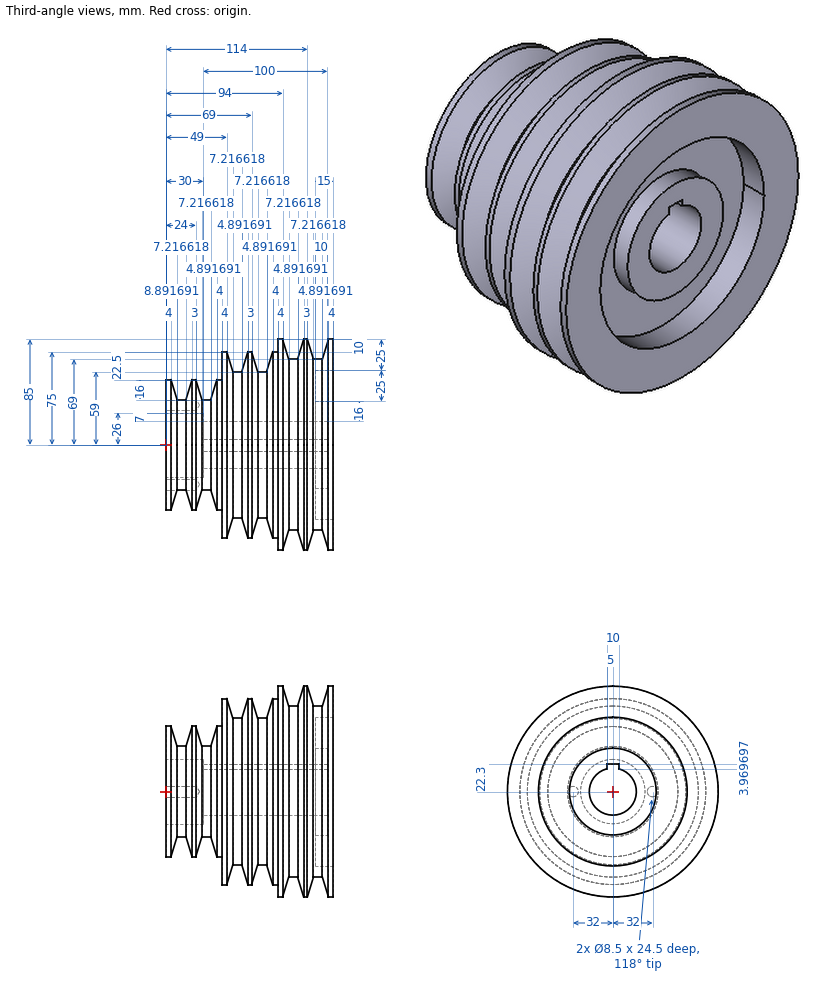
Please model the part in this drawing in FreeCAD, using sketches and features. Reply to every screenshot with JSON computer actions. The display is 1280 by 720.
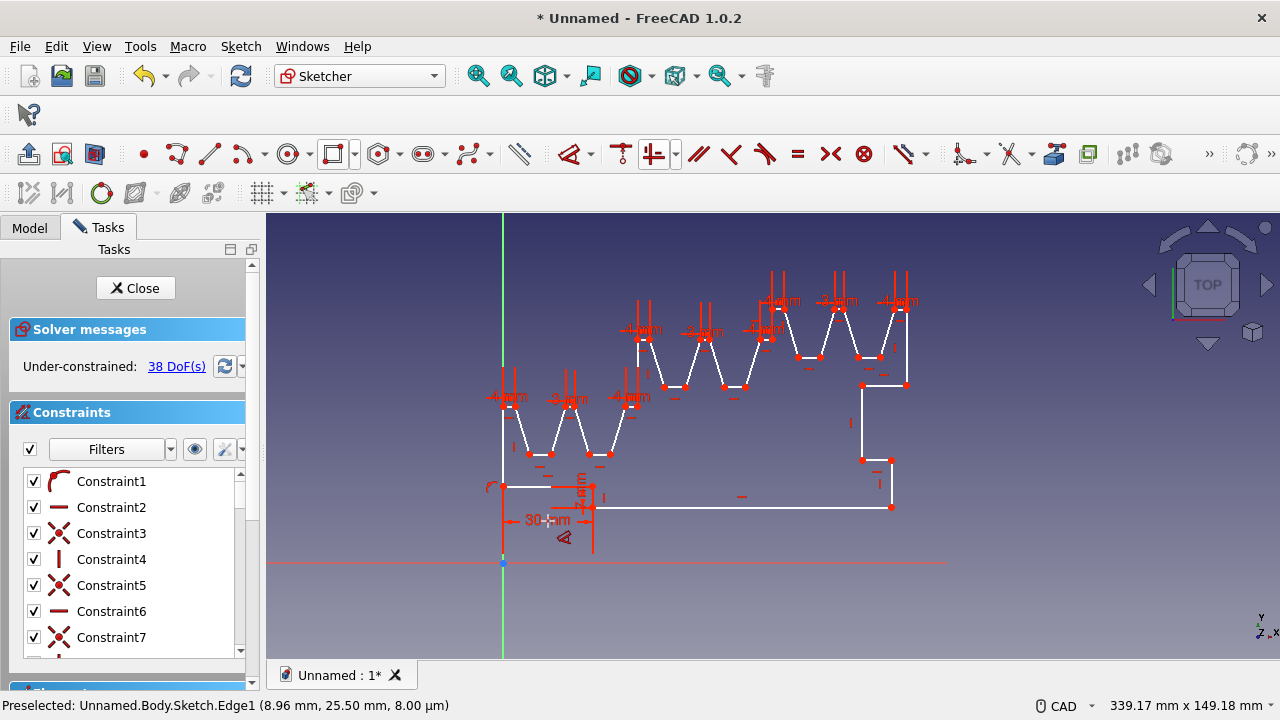
{"action": "left_click", "coordinate": [892, 494]}
{"action": "left_click", "coordinate": [926, 484]}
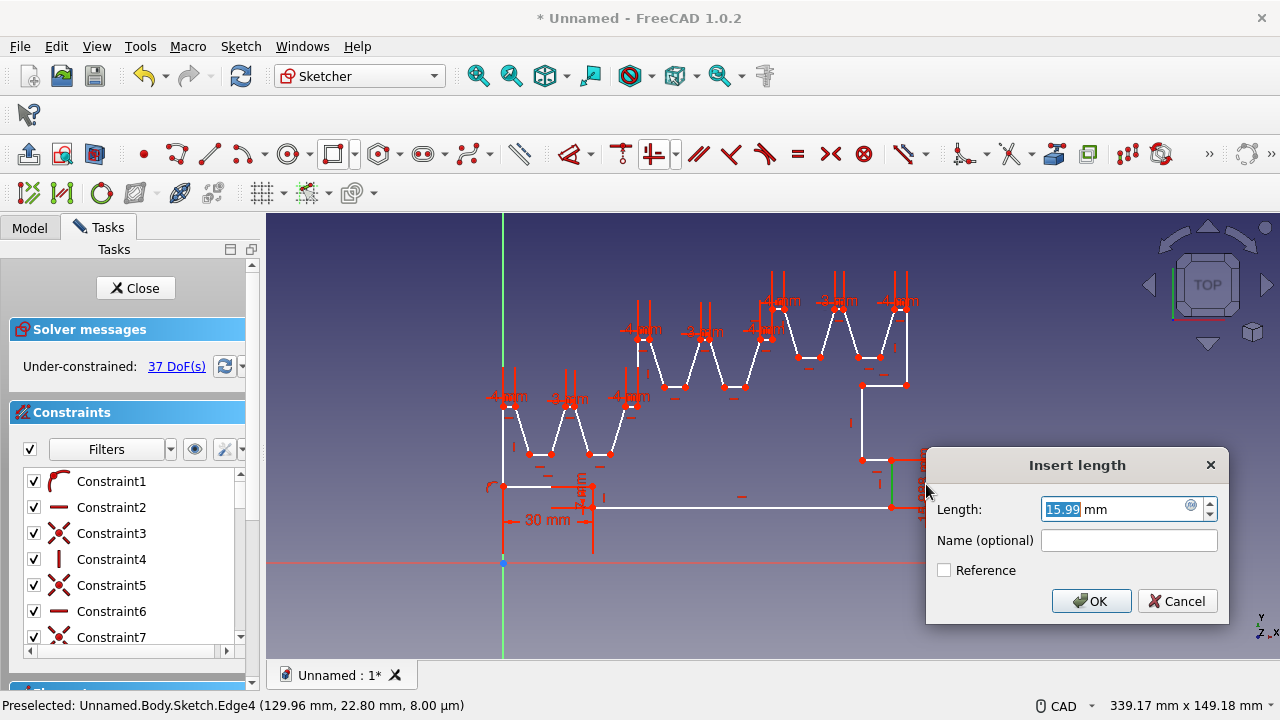
{"action": "type", "text": "16"}
{"action": "key", "text": "Return"}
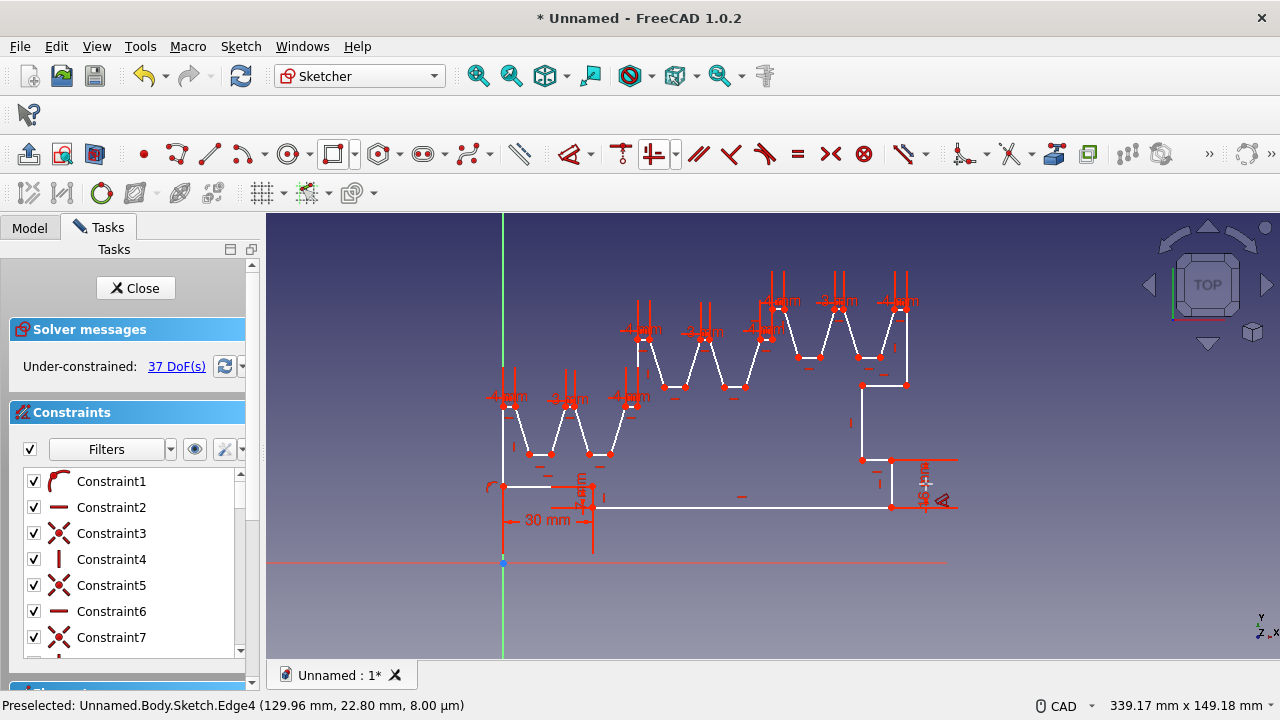
{"action": "scroll", "coordinate": [880, 460], "scroll_direction": "up", "scroll_amount": 2}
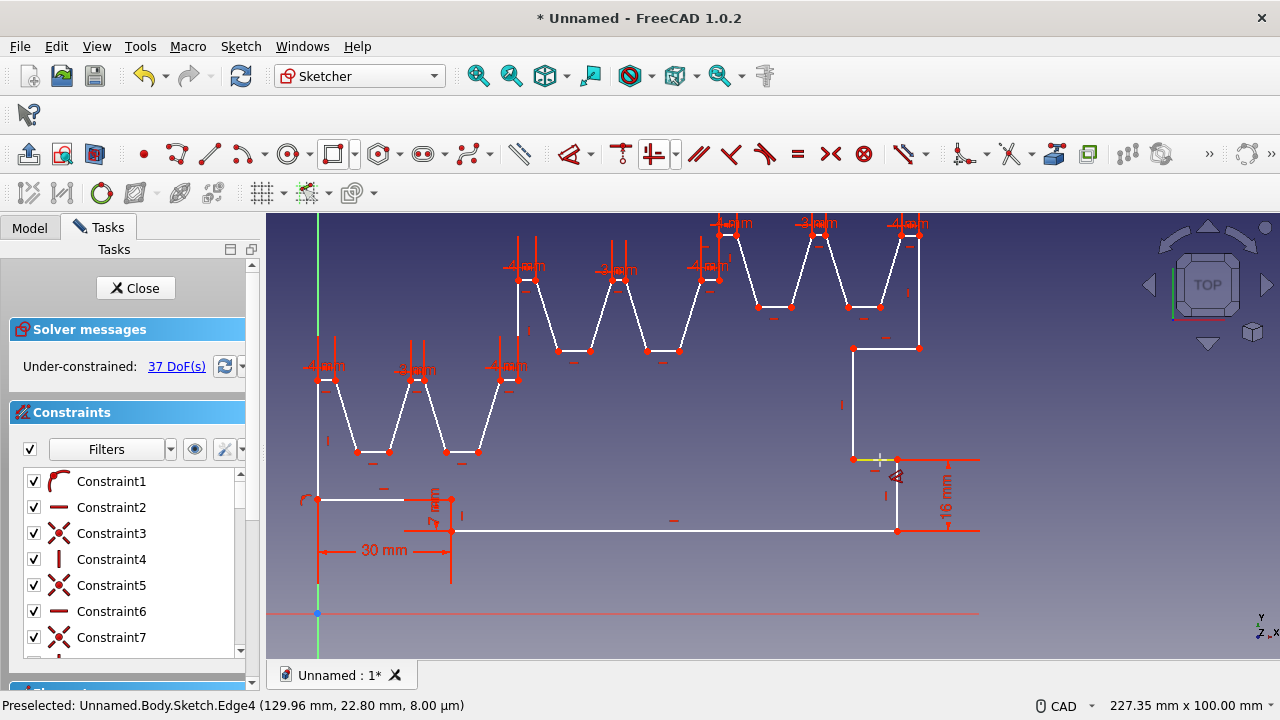
{"action": "left_click", "coordinate": [880, 460]}
{"action": "left_click", "coordinate": [875, 494]}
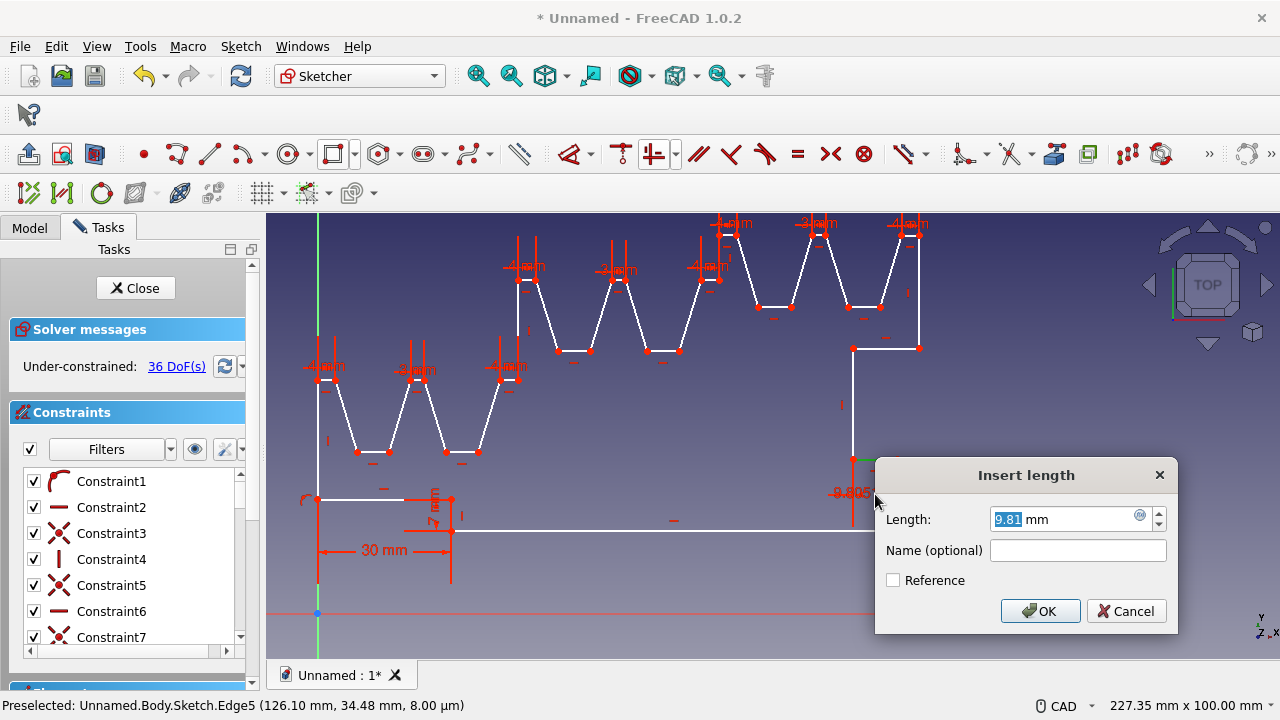
{"action": "type", "text": "10"}
{"action": "key", "text": "Return"}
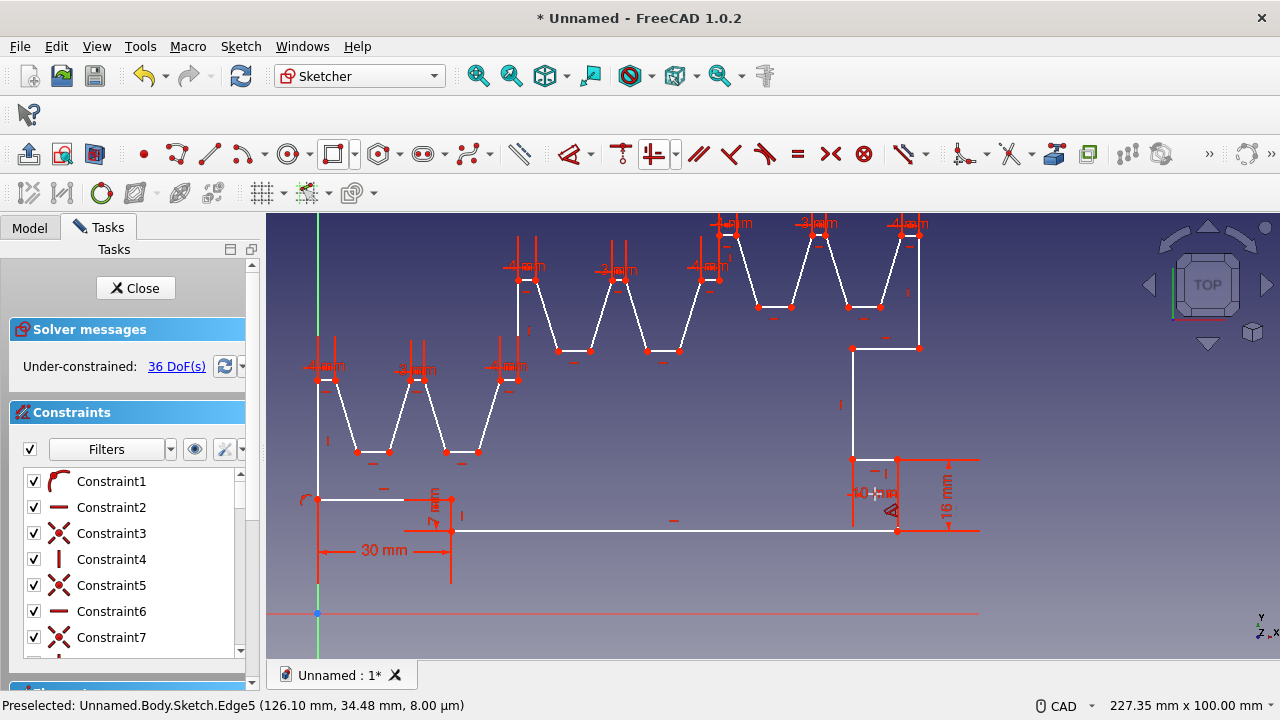
{"action": "left_click", "coordinate": [853, 426]}
{"action": "left_click", "coordinate": [887, 404]}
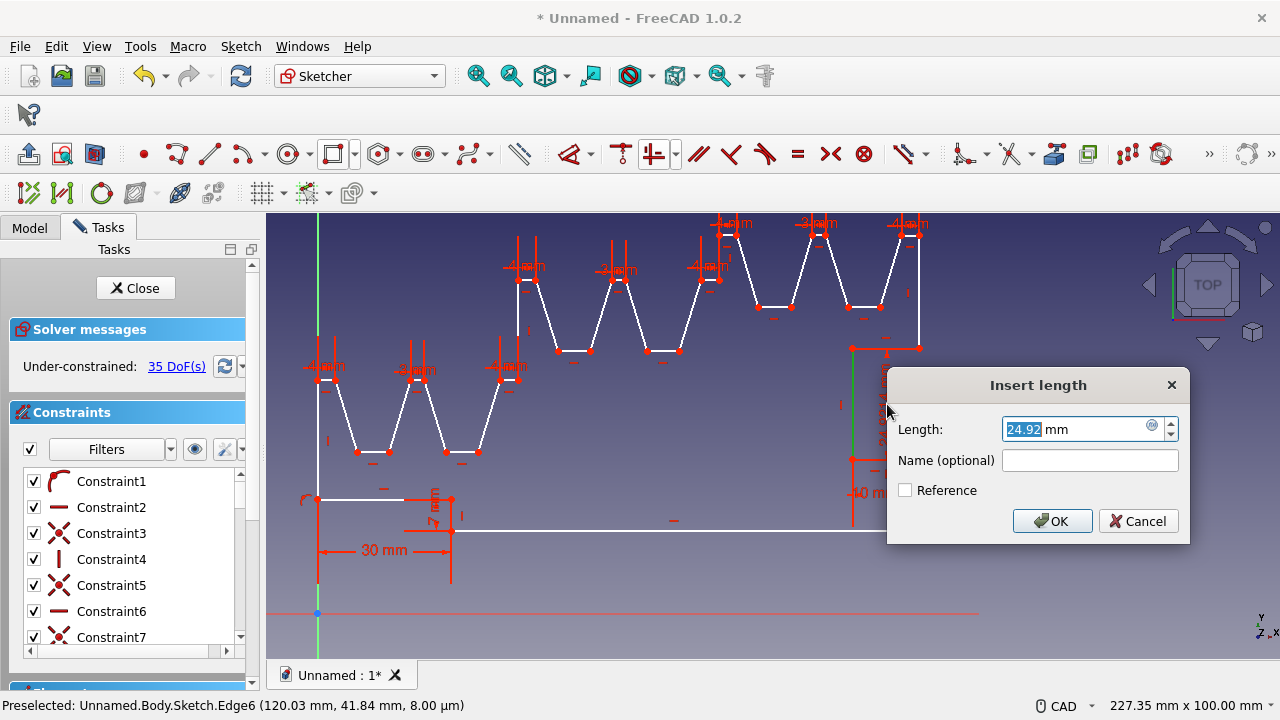
{"action": "type", "text": "25"}
{"action": "key", "text": "Return"}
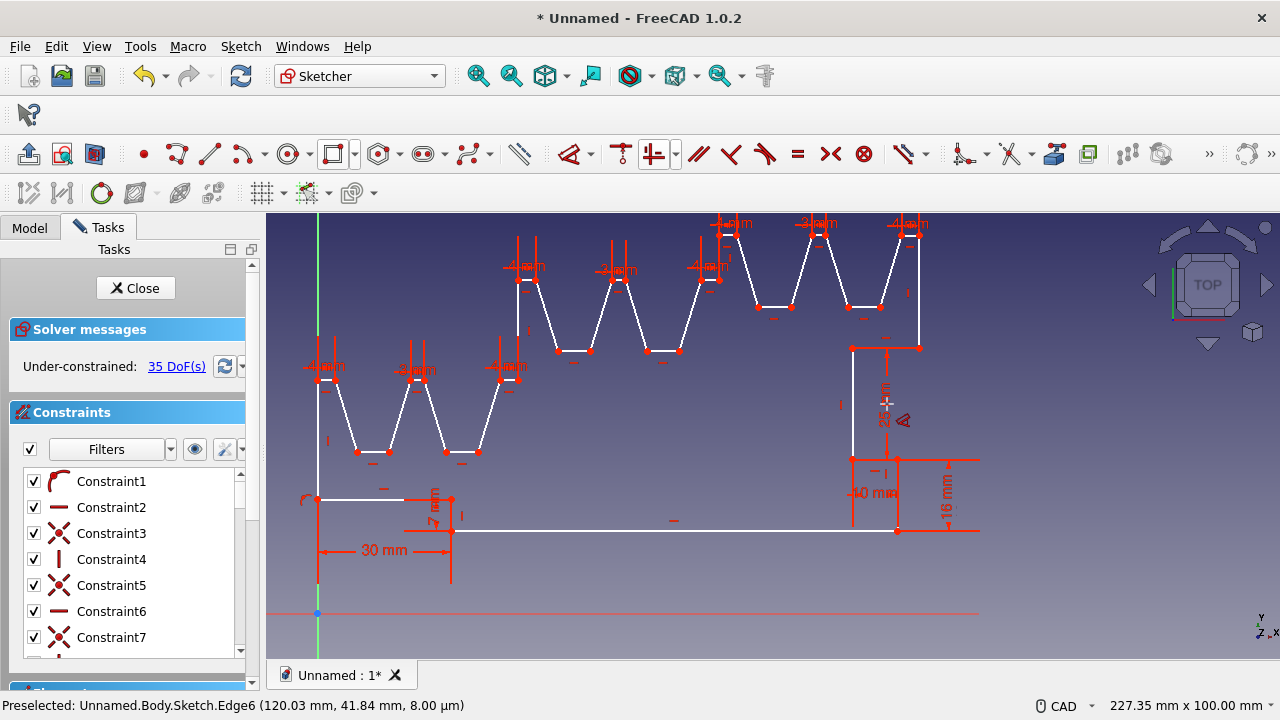
{"action": "left_click", "coordinate": [873, 348]}
{"action": "left_click", "coordinate": [901, 314]}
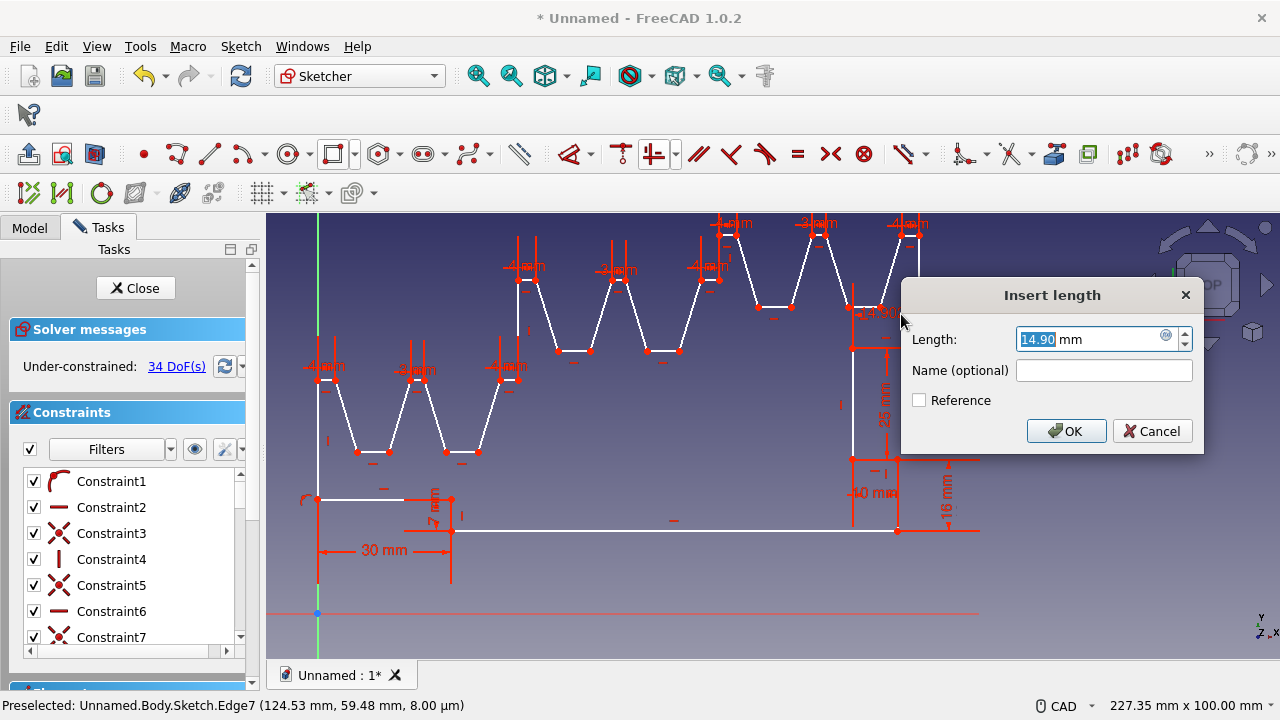
{"action": "type", "text": "15"}
{"action": "key", "text": "Return"}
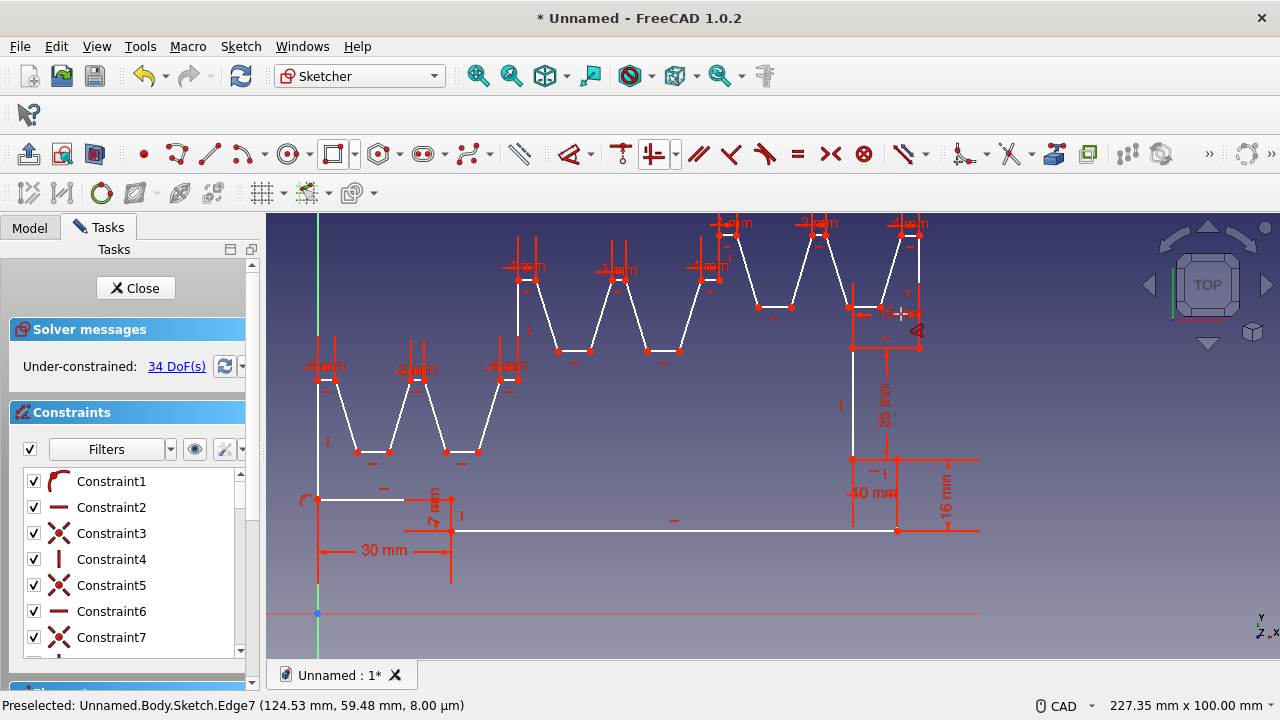
{"action": "left_click", "coordinate": [919, 315]}
{"action": "left_click", "coordinate": [953, 270]}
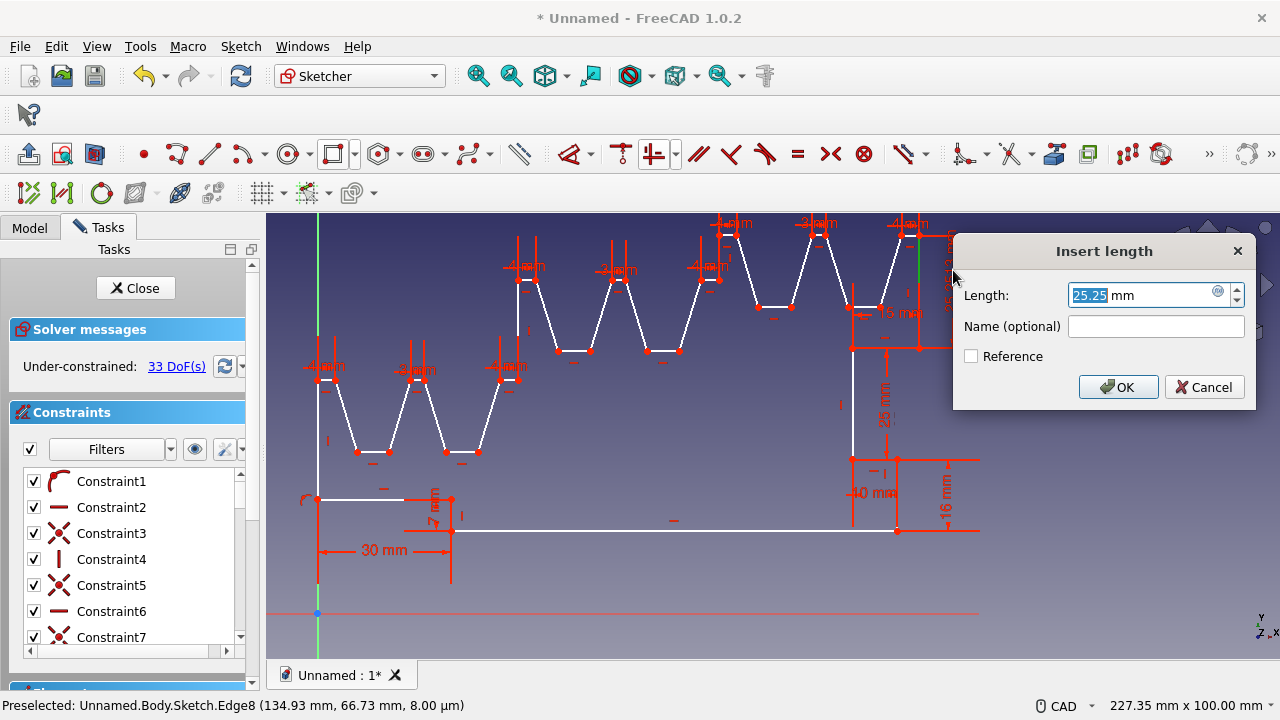
{"action": "type", "text": "25"}
{"action": "key", "text": "Return"}